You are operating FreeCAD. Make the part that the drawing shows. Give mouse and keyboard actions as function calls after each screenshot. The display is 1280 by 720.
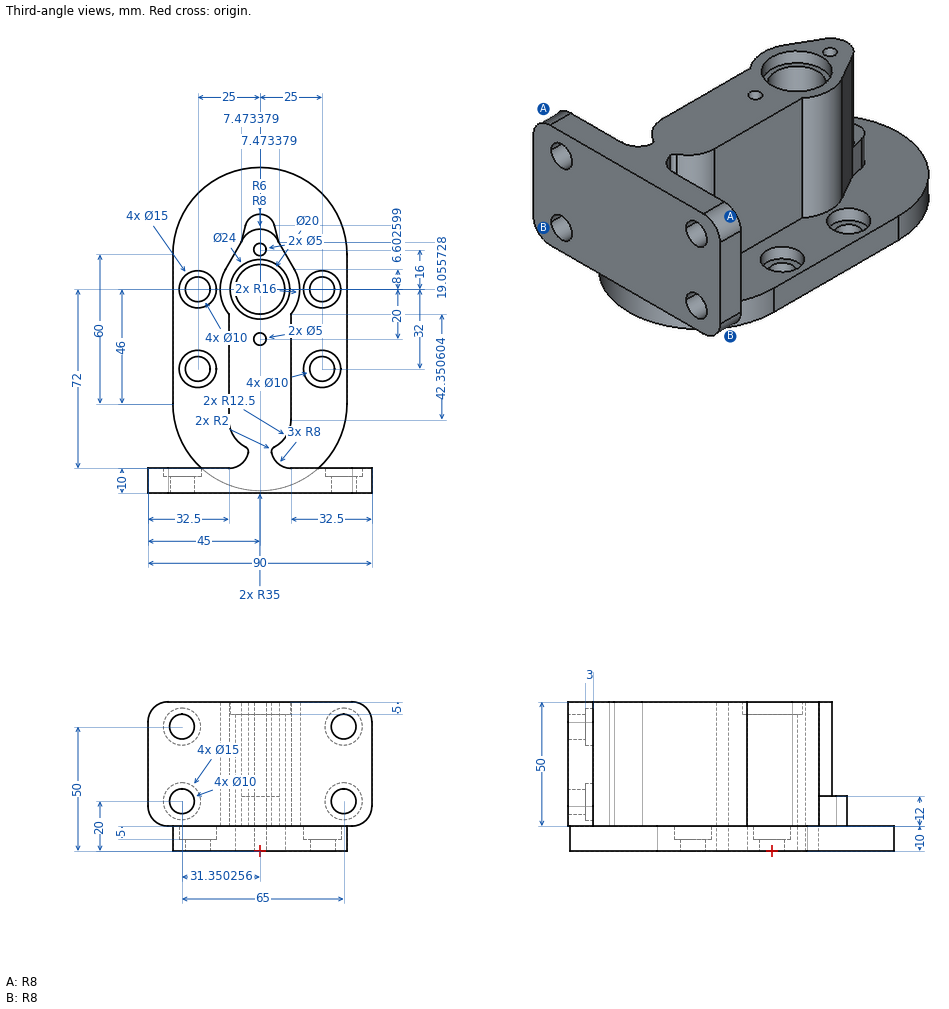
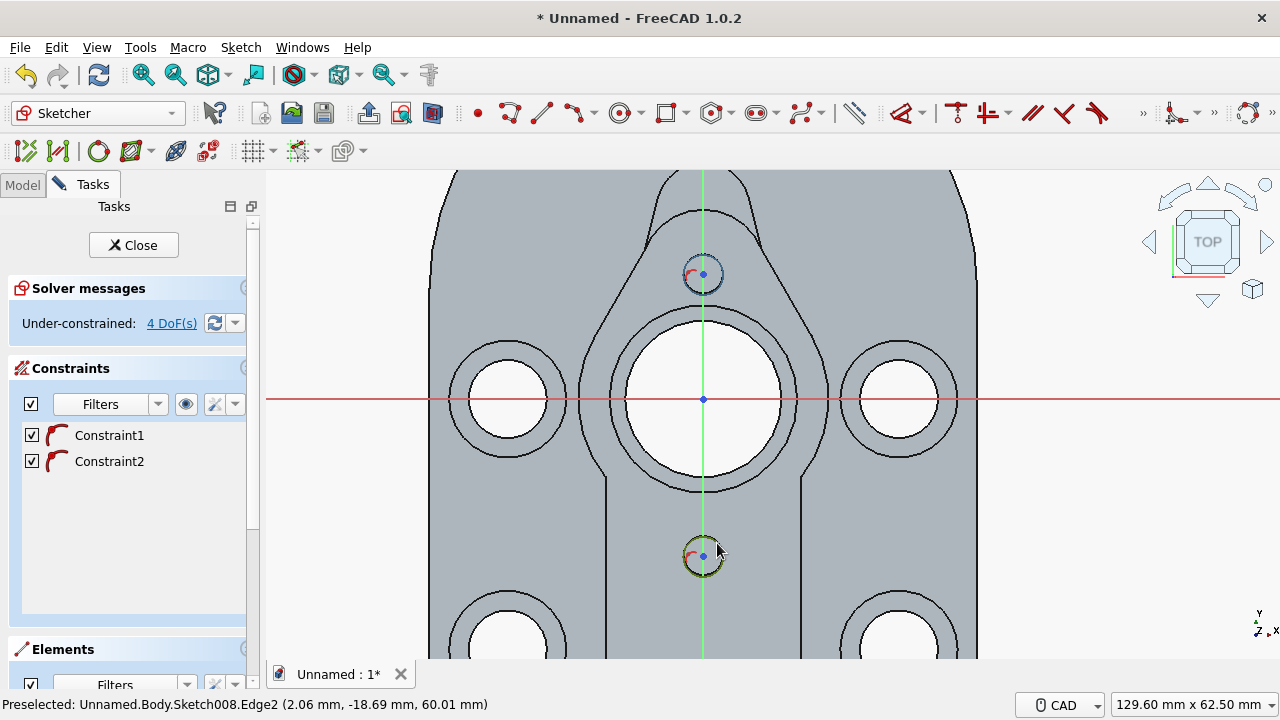
key(e)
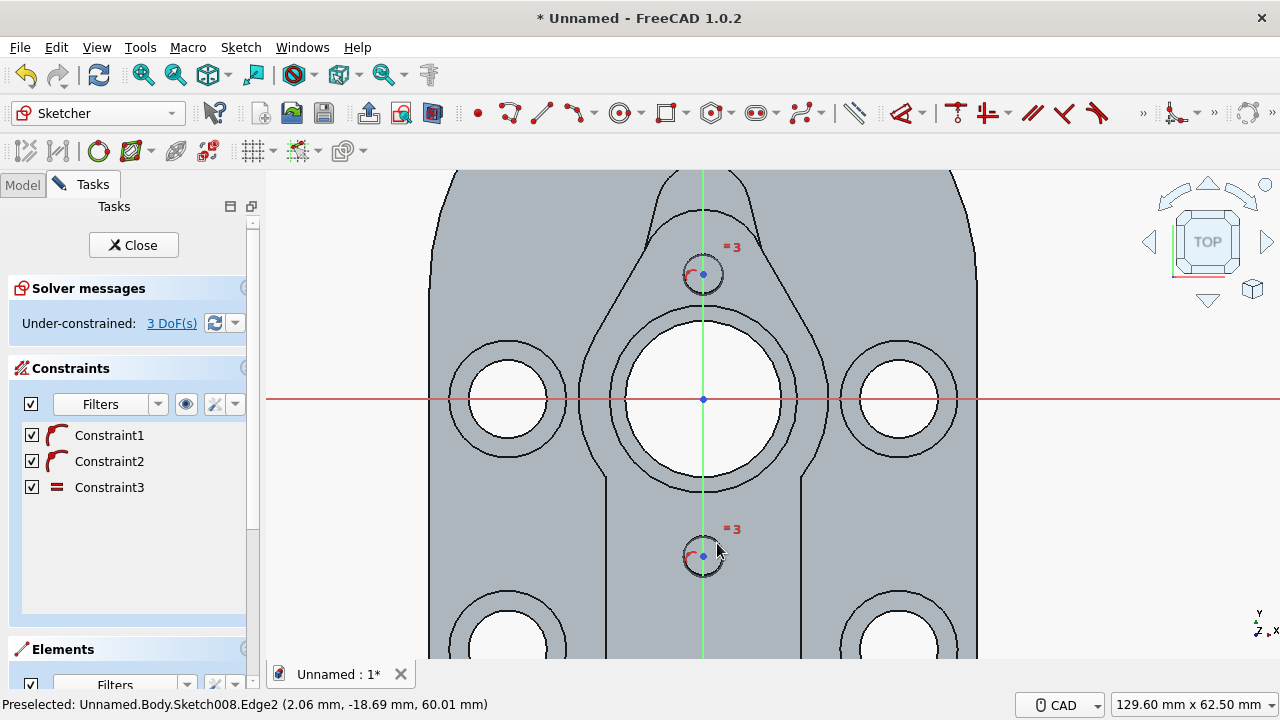
click(902, 114)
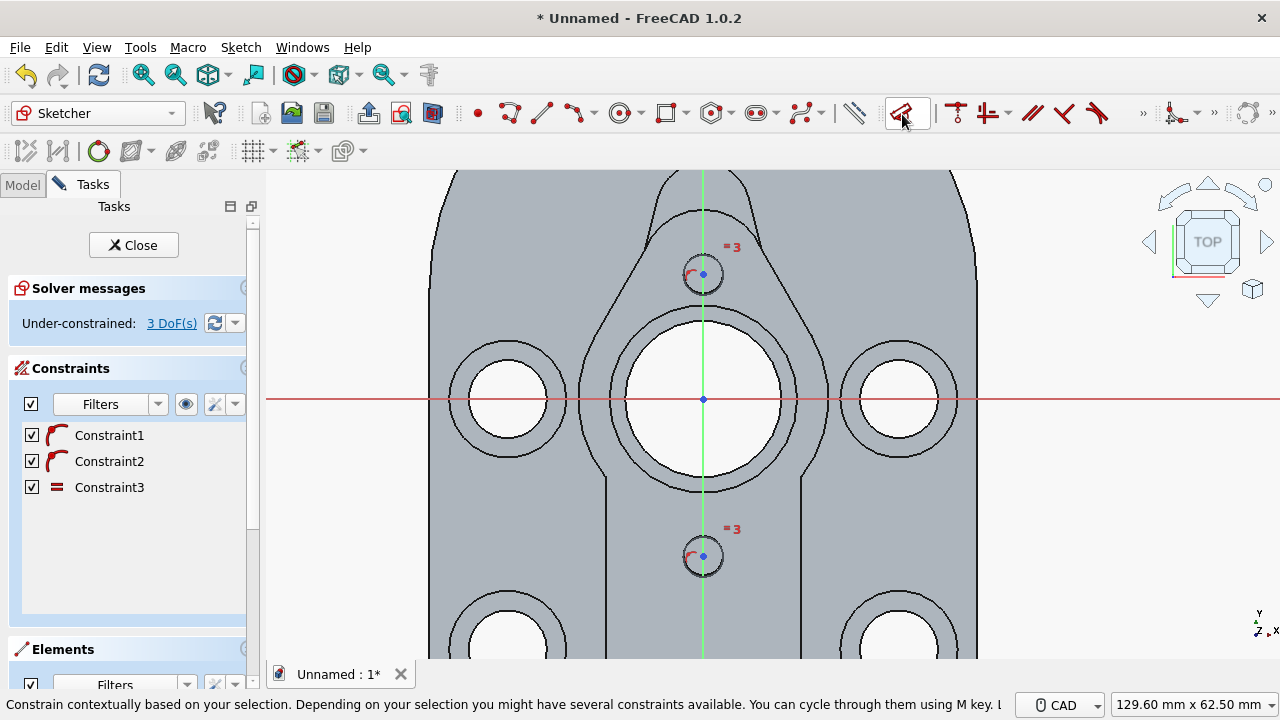
click(717, 261)
click(739, 238)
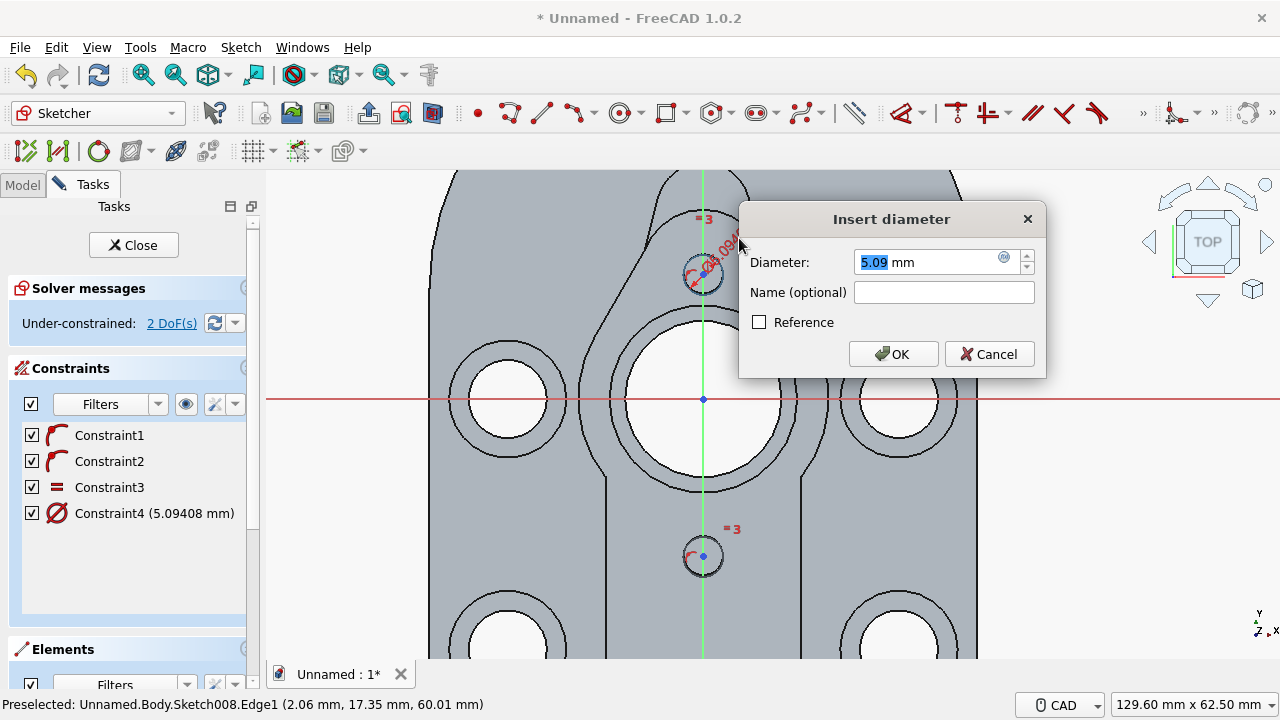
text(5)
key(Return)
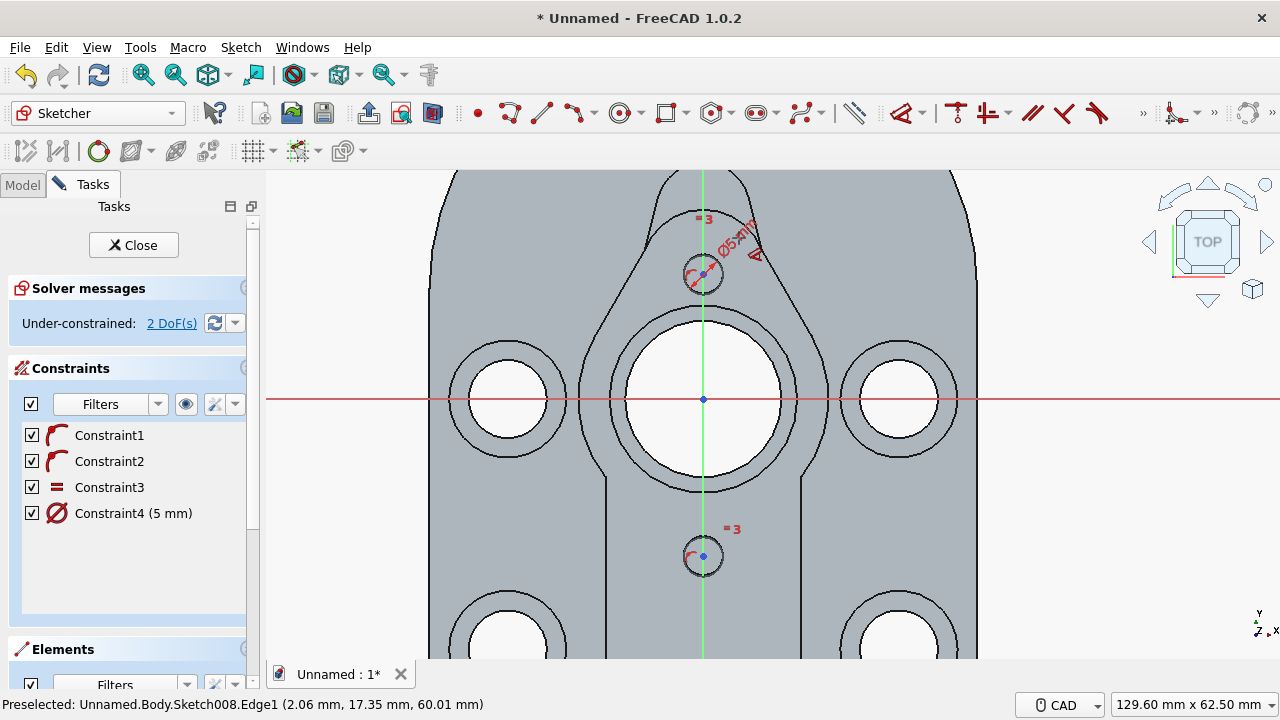
click(703, 275)
click(737, 337)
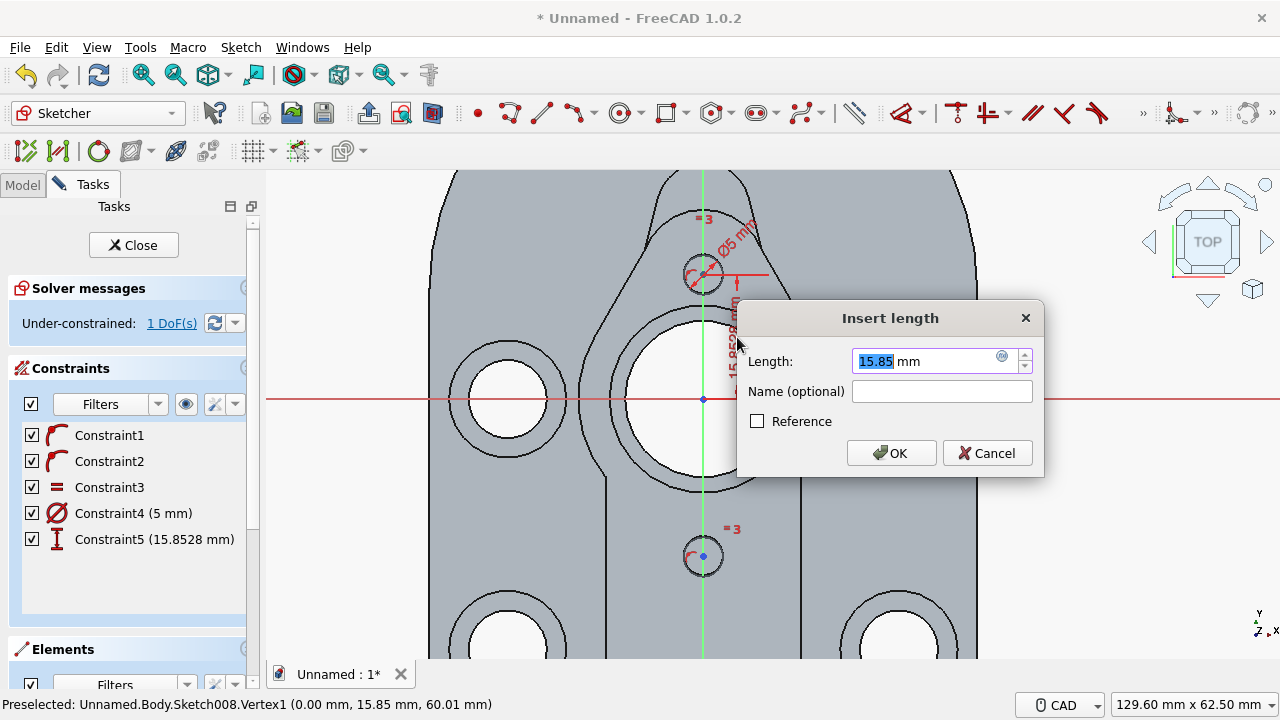
text(16)
key(Return)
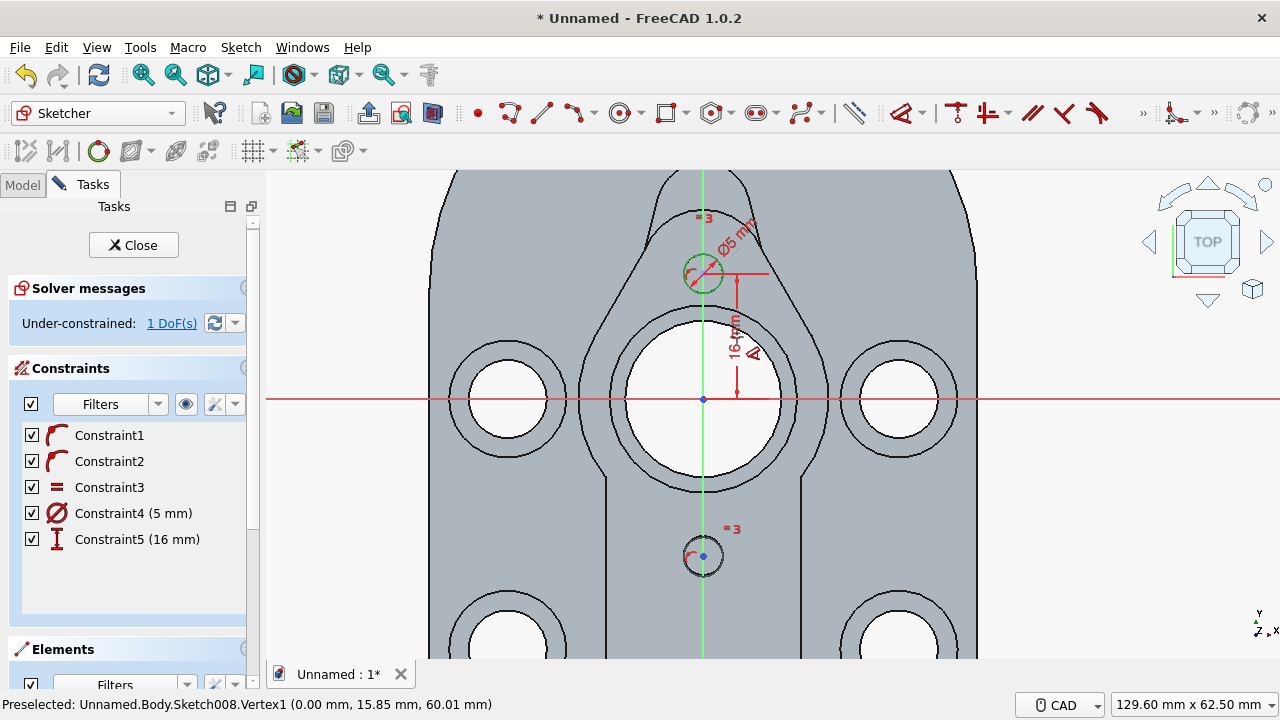
click(703, 557)
click(737, 478)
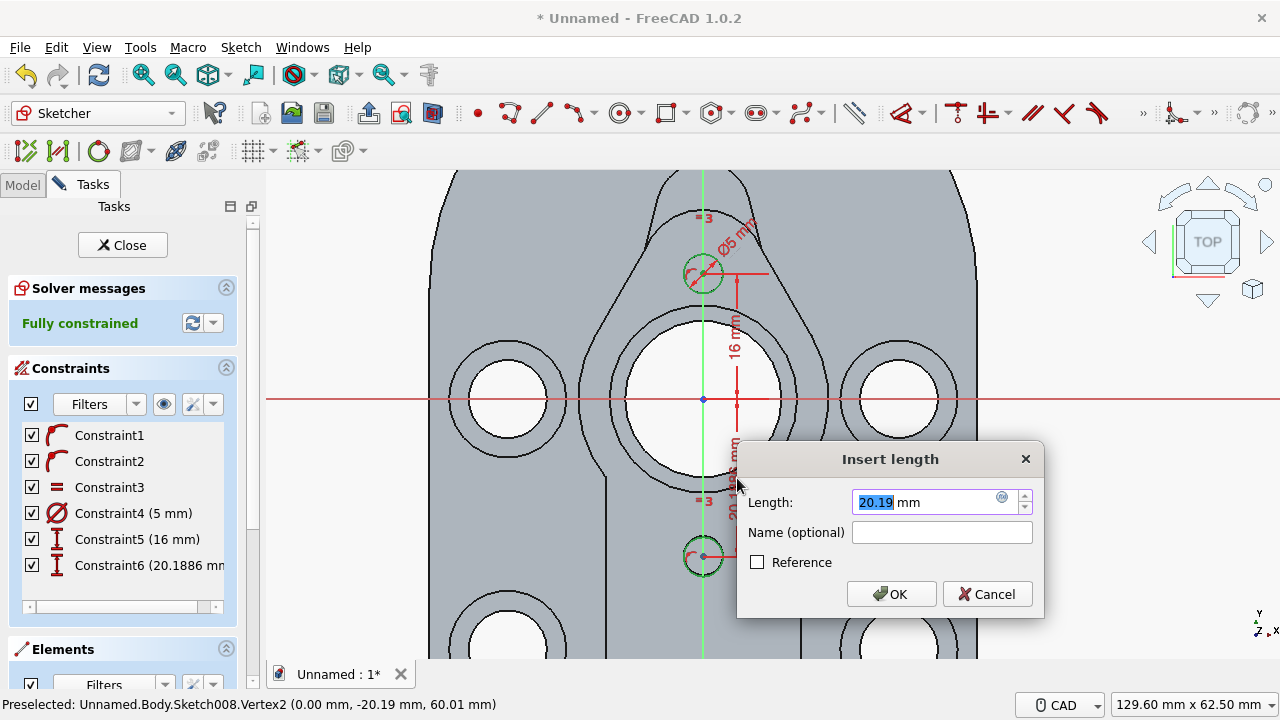
text(20)
key(Return)
key(Escape)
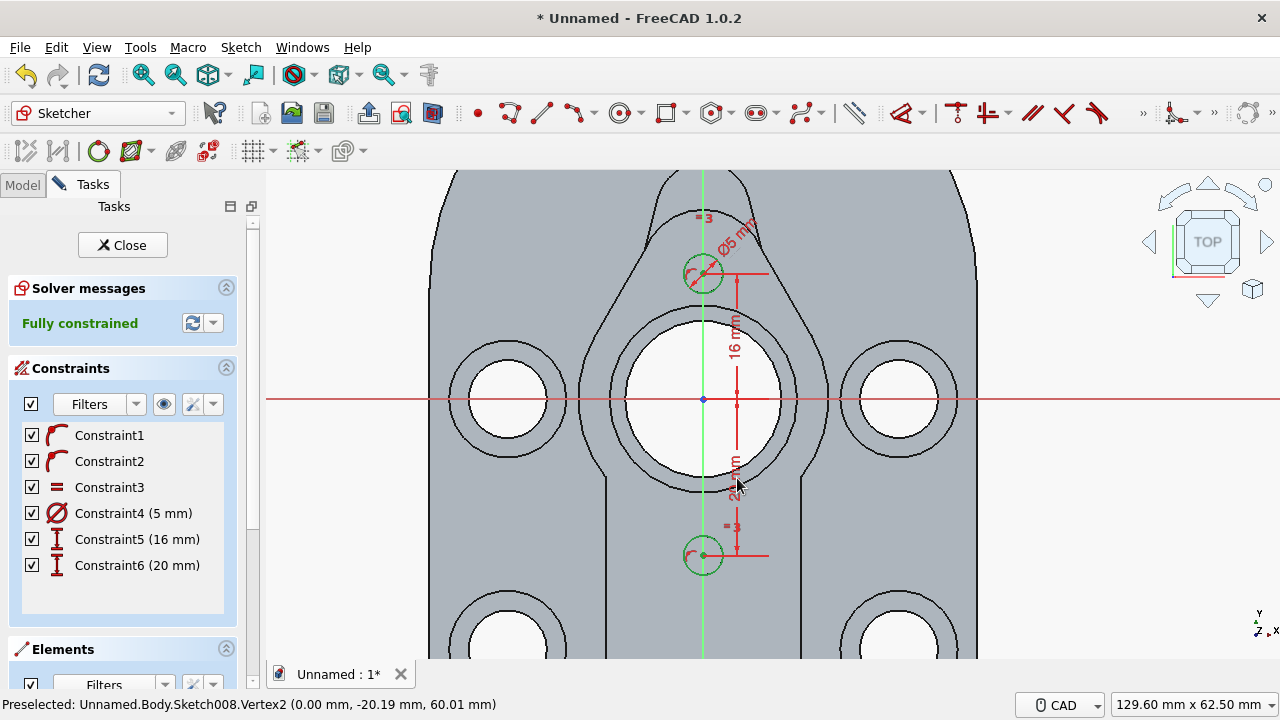
click(123, 245)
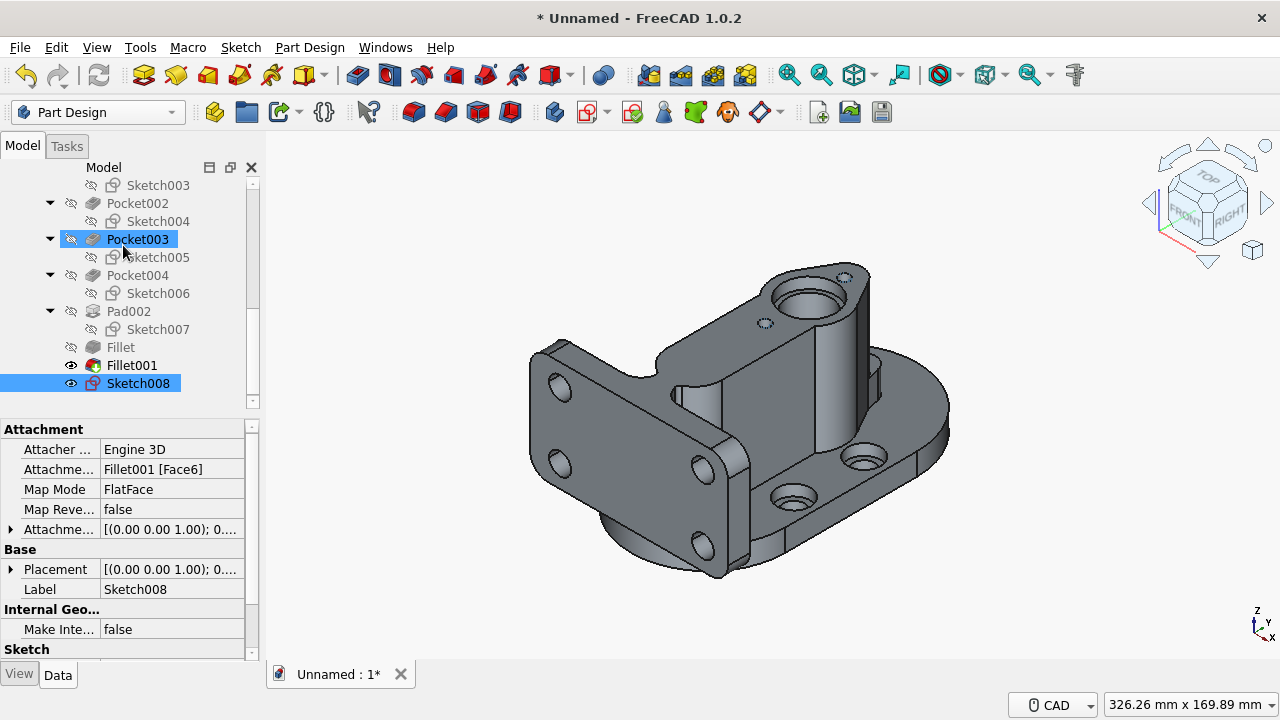
click(358, 76)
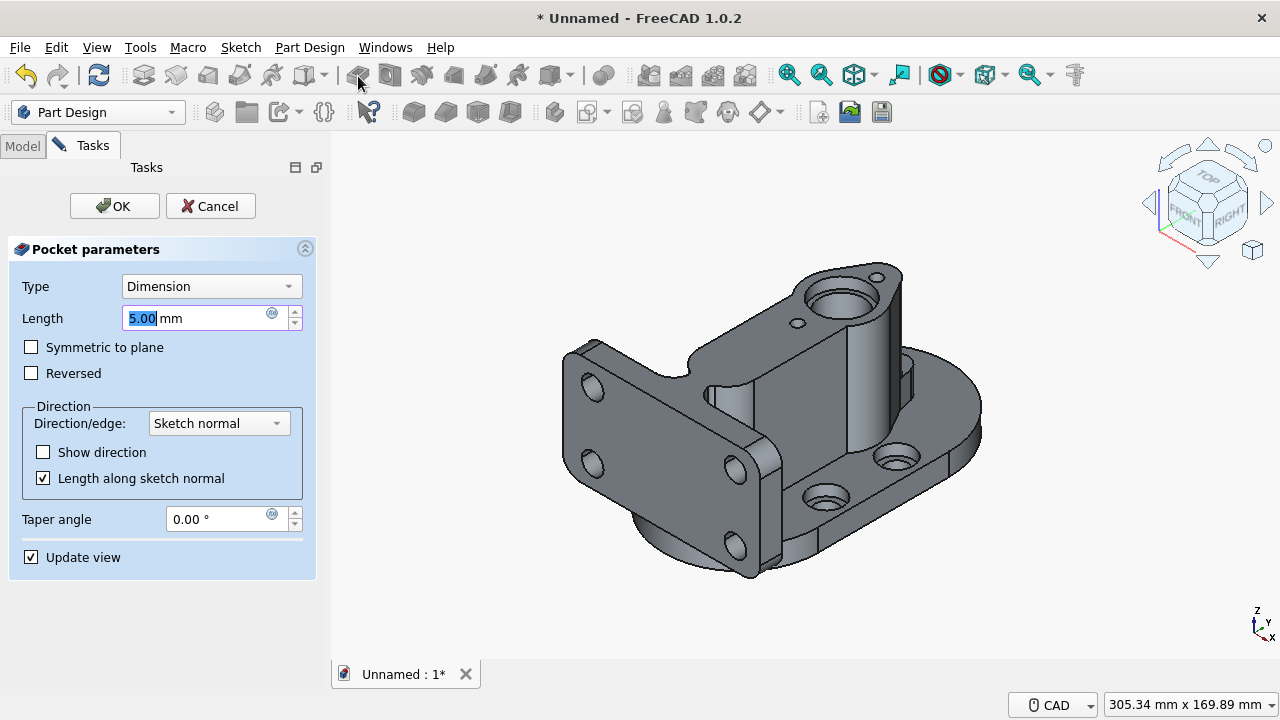
click(212, 286)